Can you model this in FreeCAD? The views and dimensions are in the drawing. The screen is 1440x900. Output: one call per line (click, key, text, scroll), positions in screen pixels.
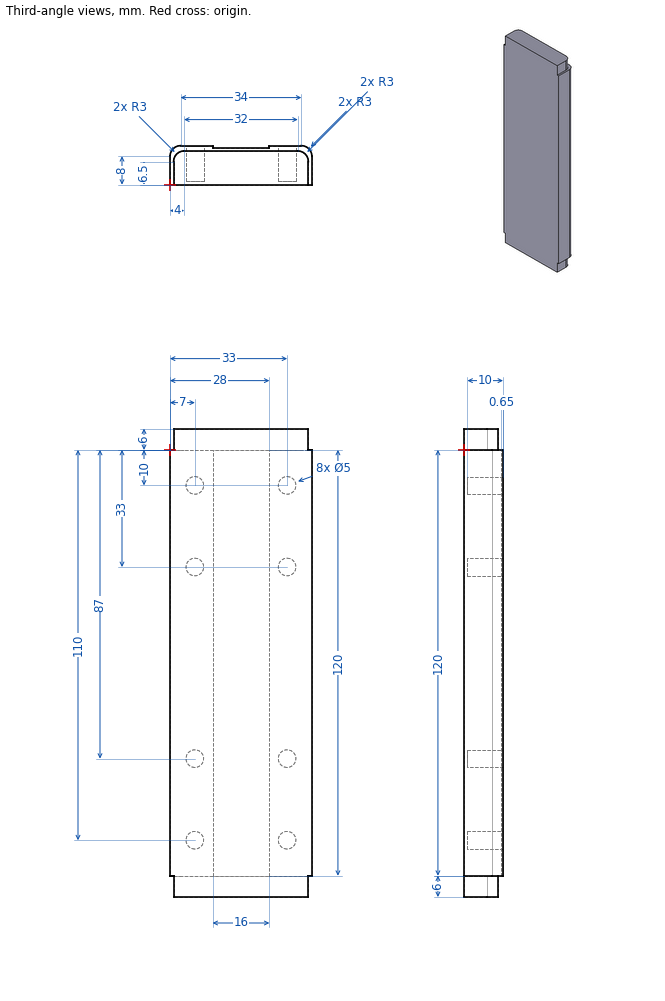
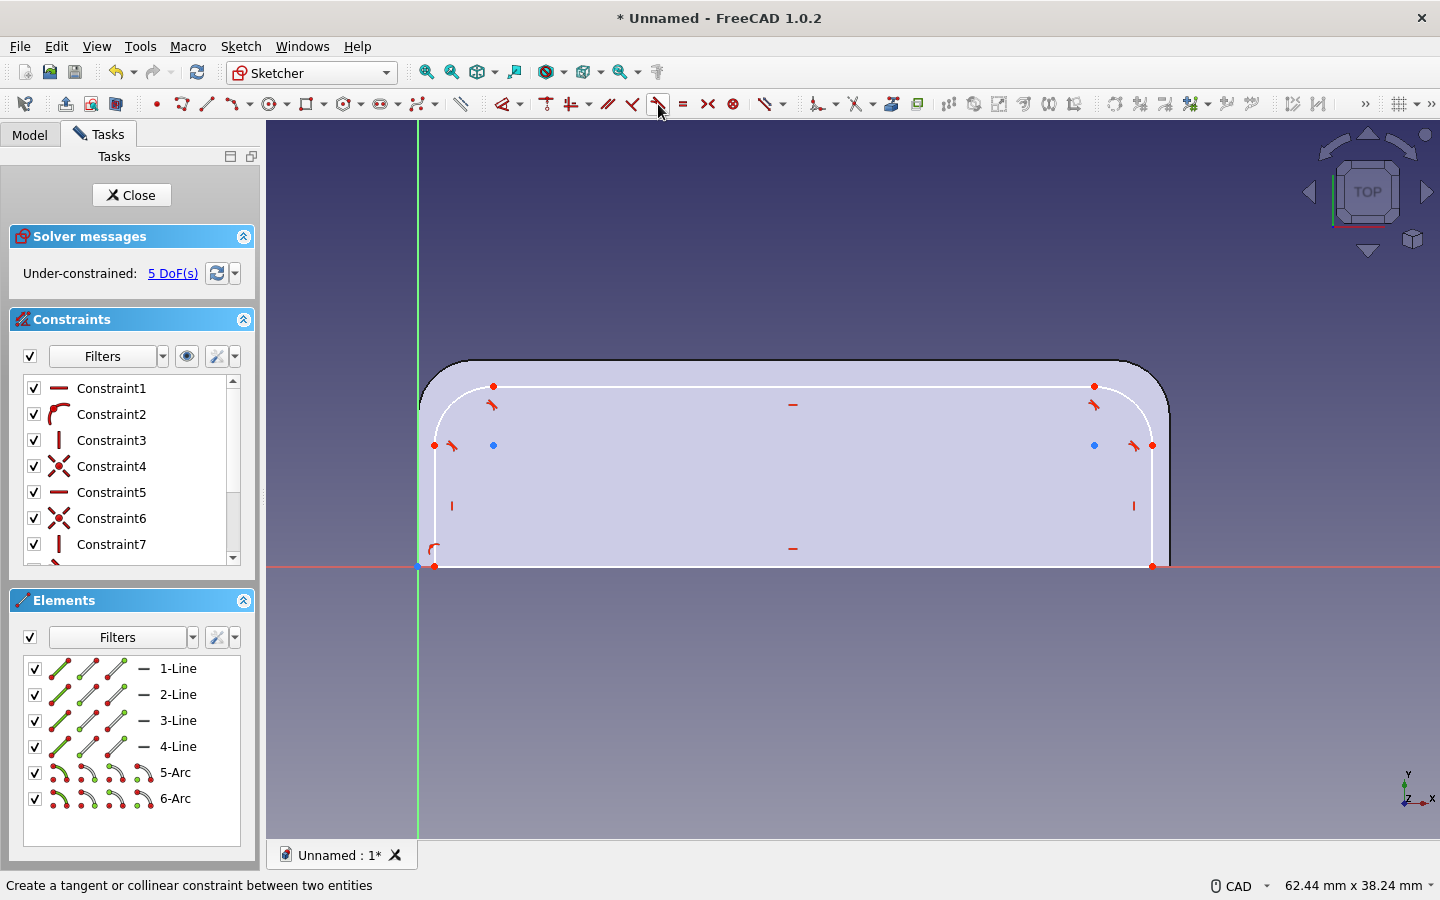
click(467, 393)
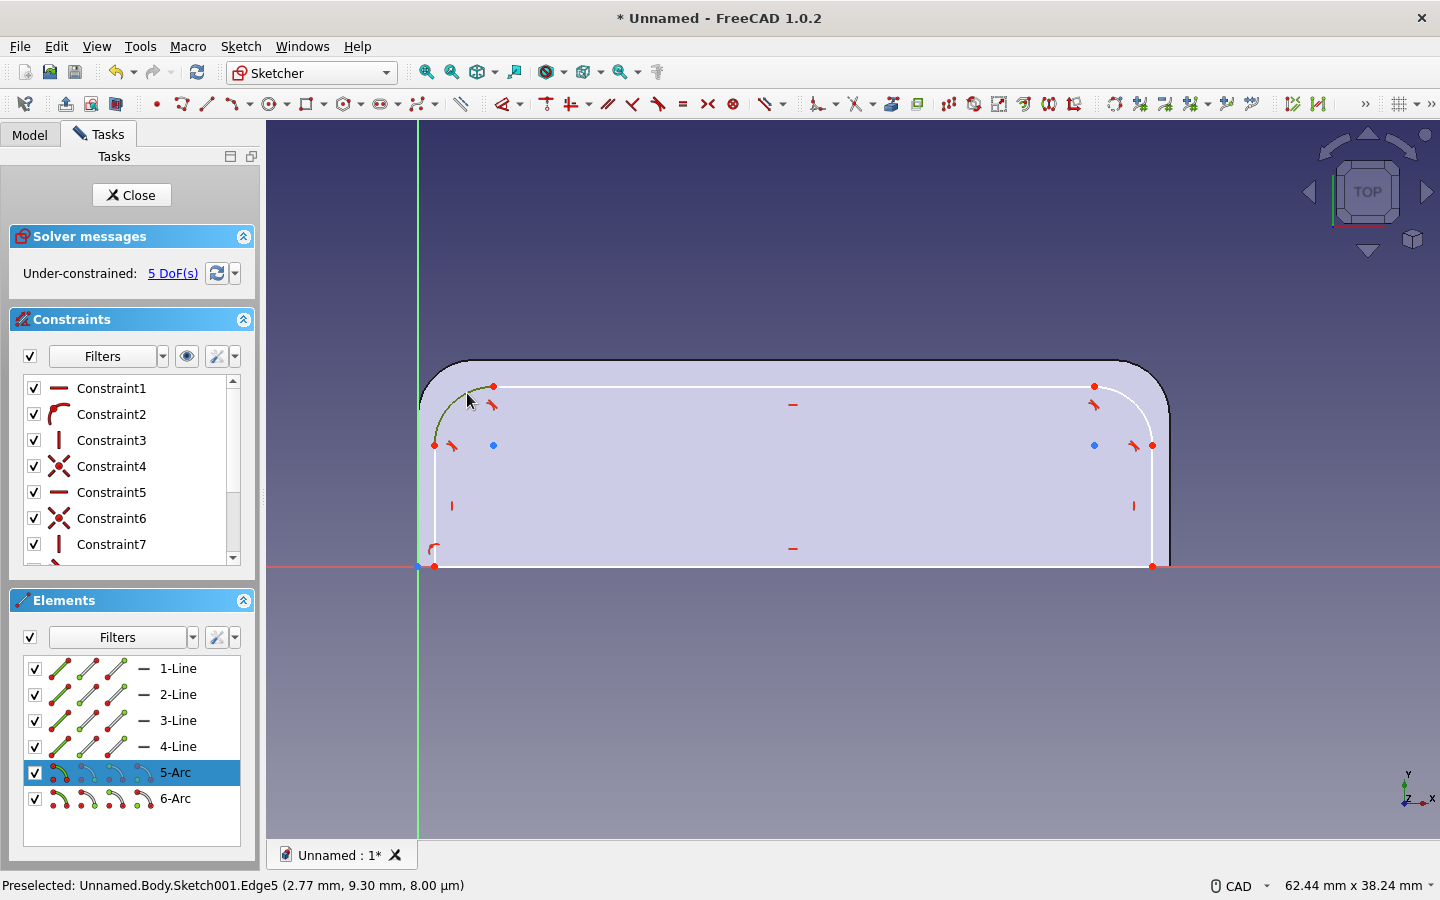
click(1146, 419)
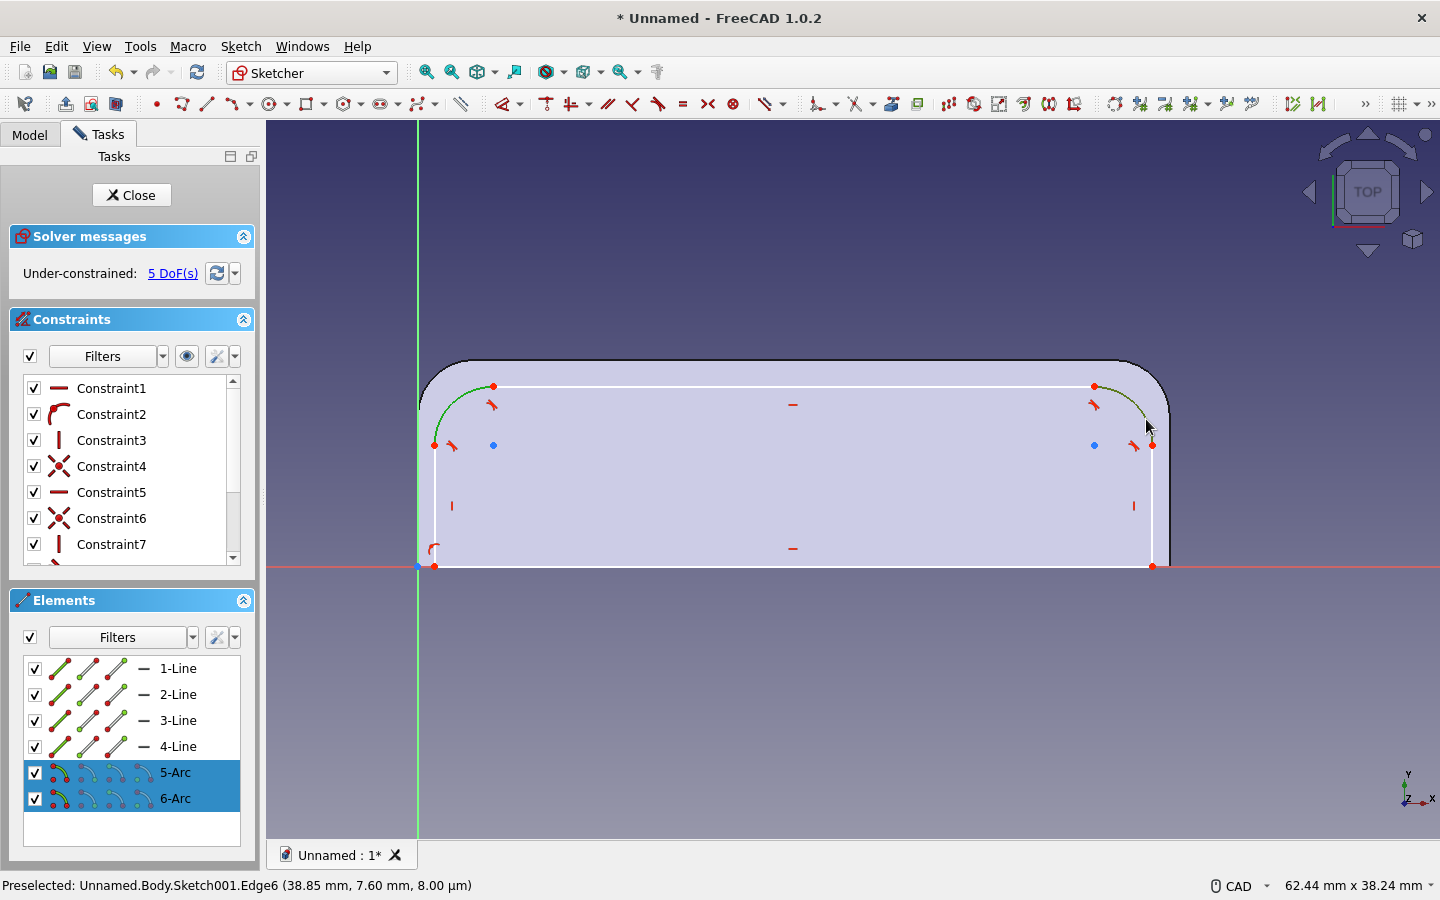
click(683, 104)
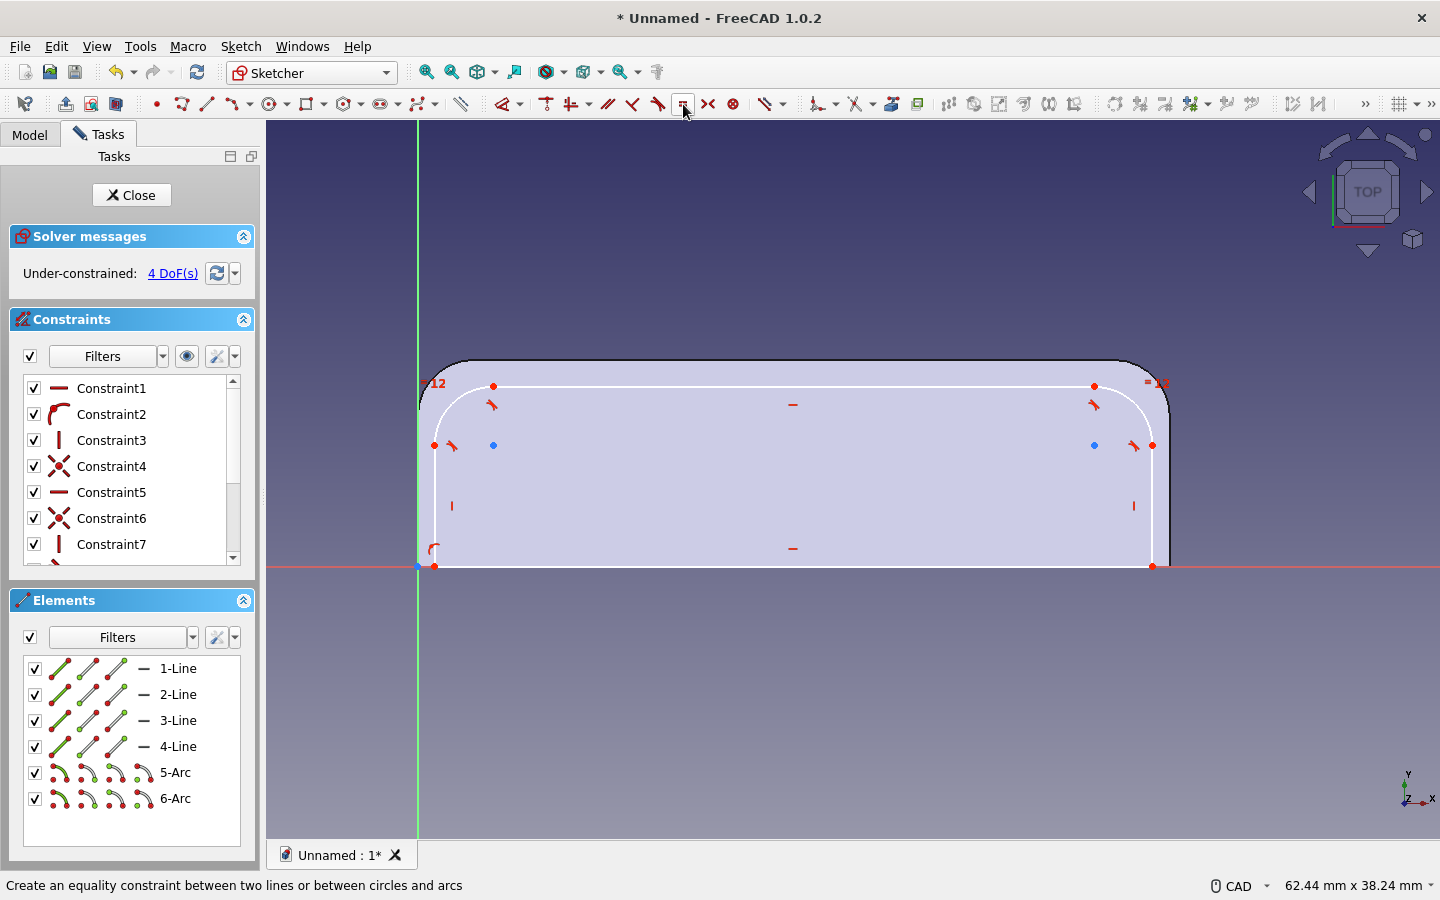
key(d)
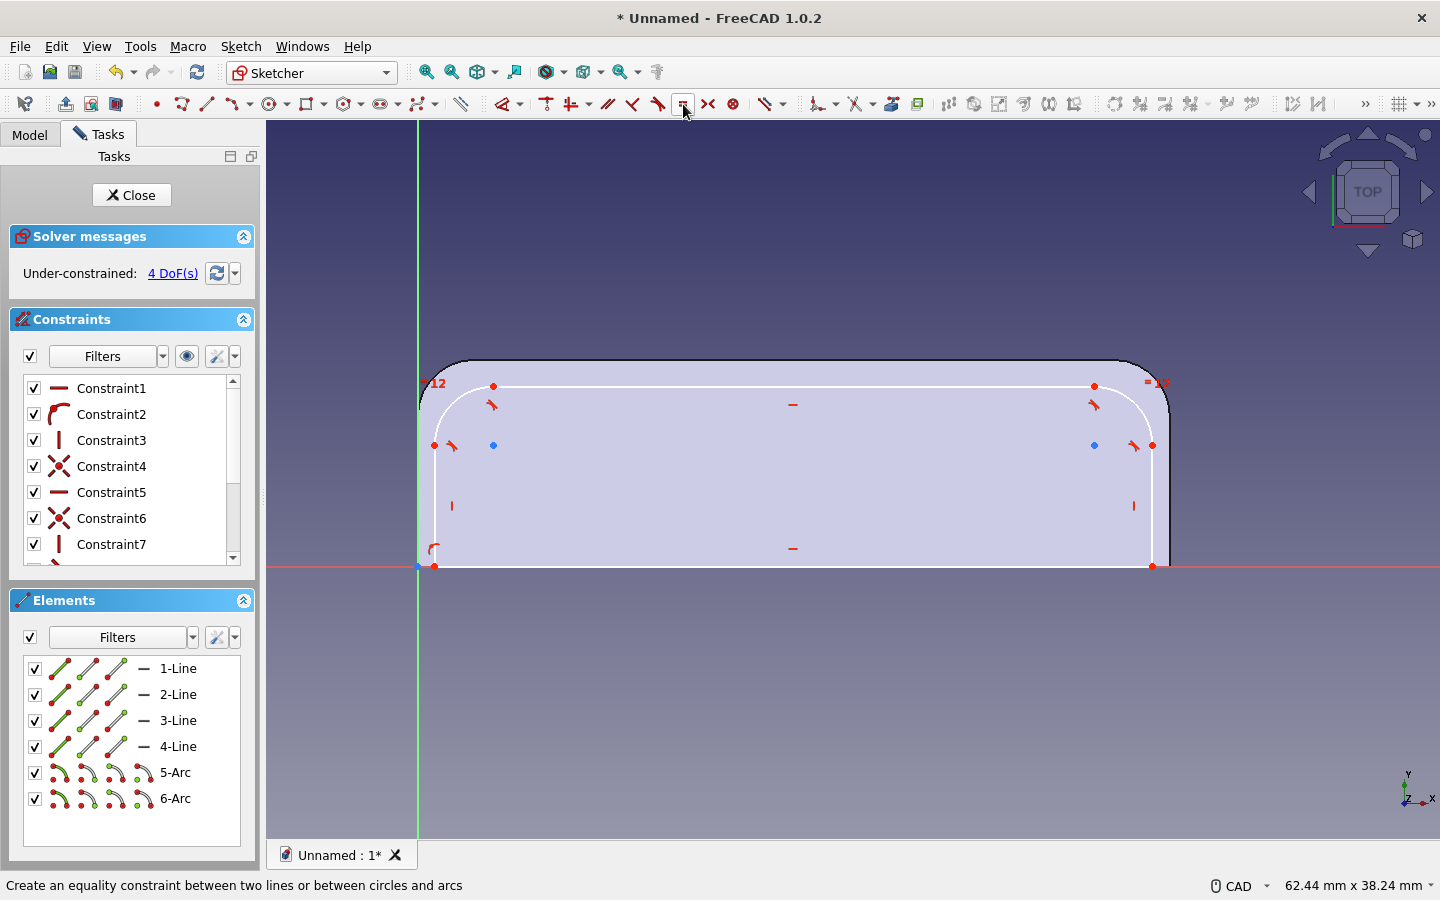
click(467, 393)
click(453, 364)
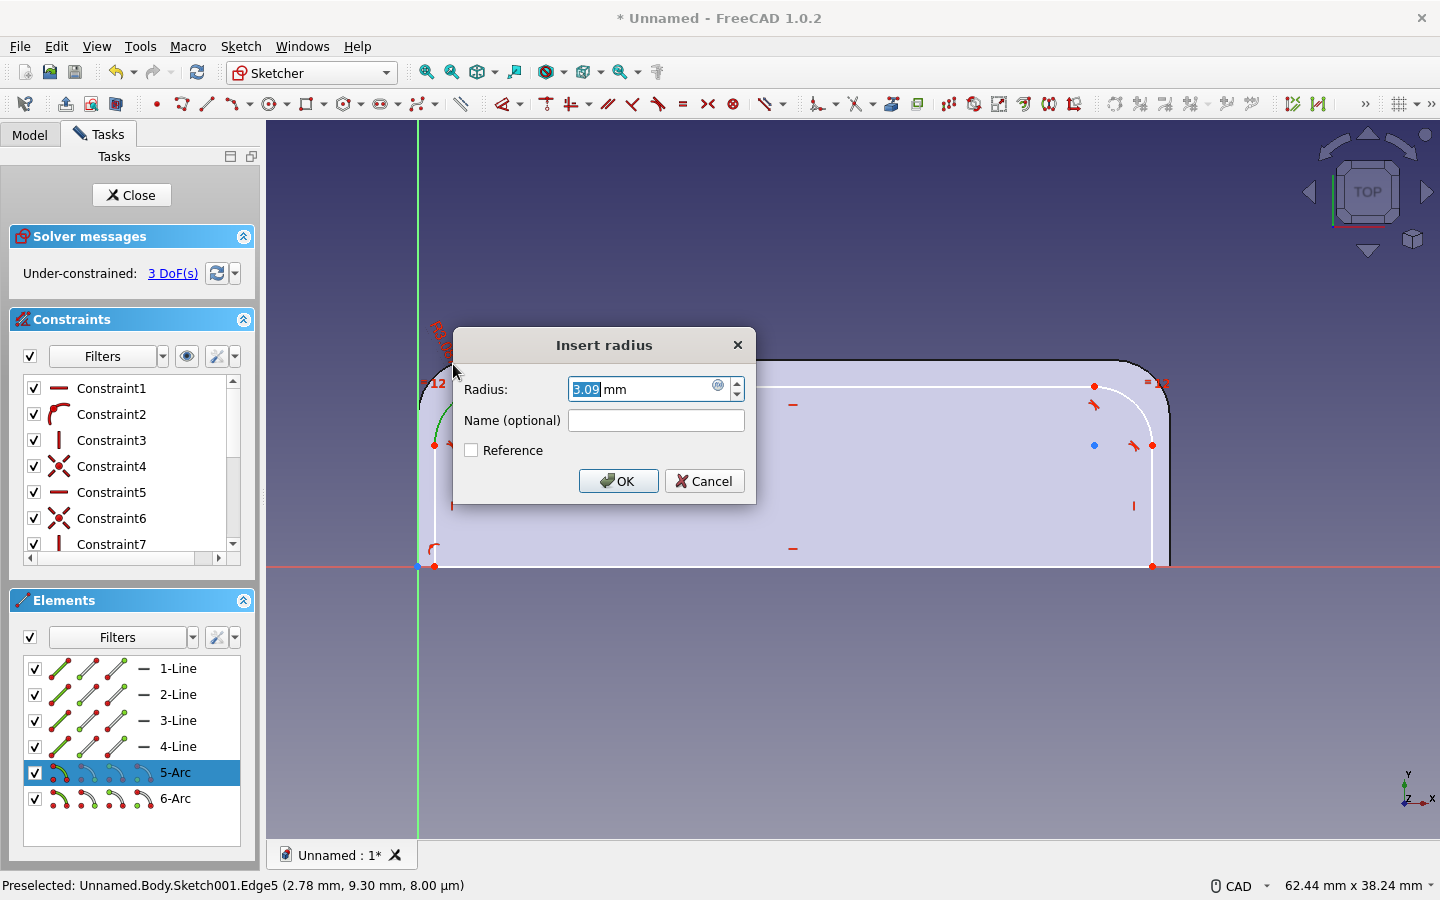
text(3)
key(Return)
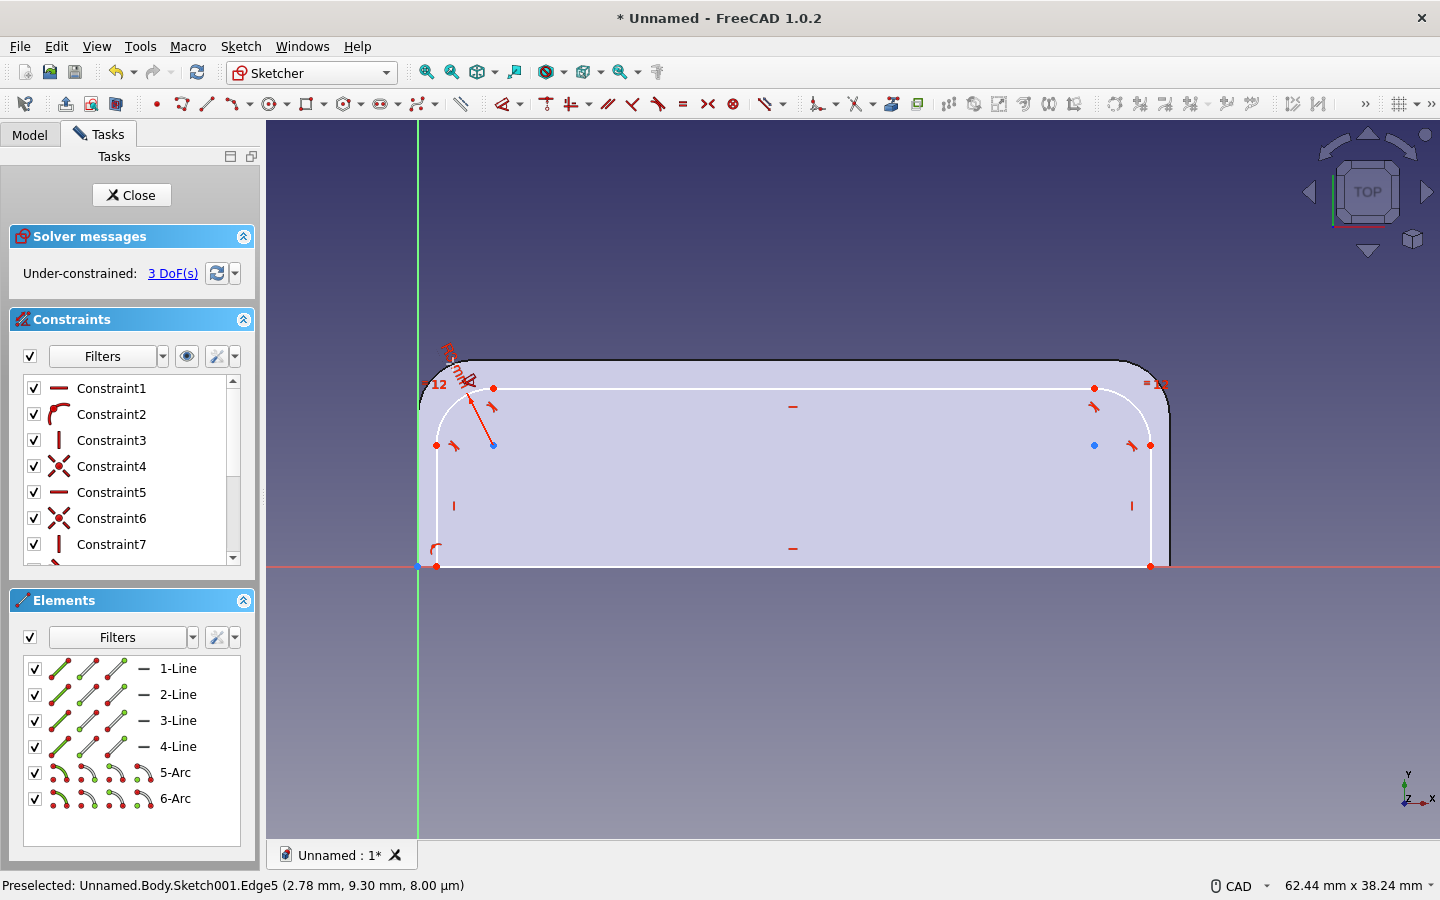
click(914, 389)
click(794, 355)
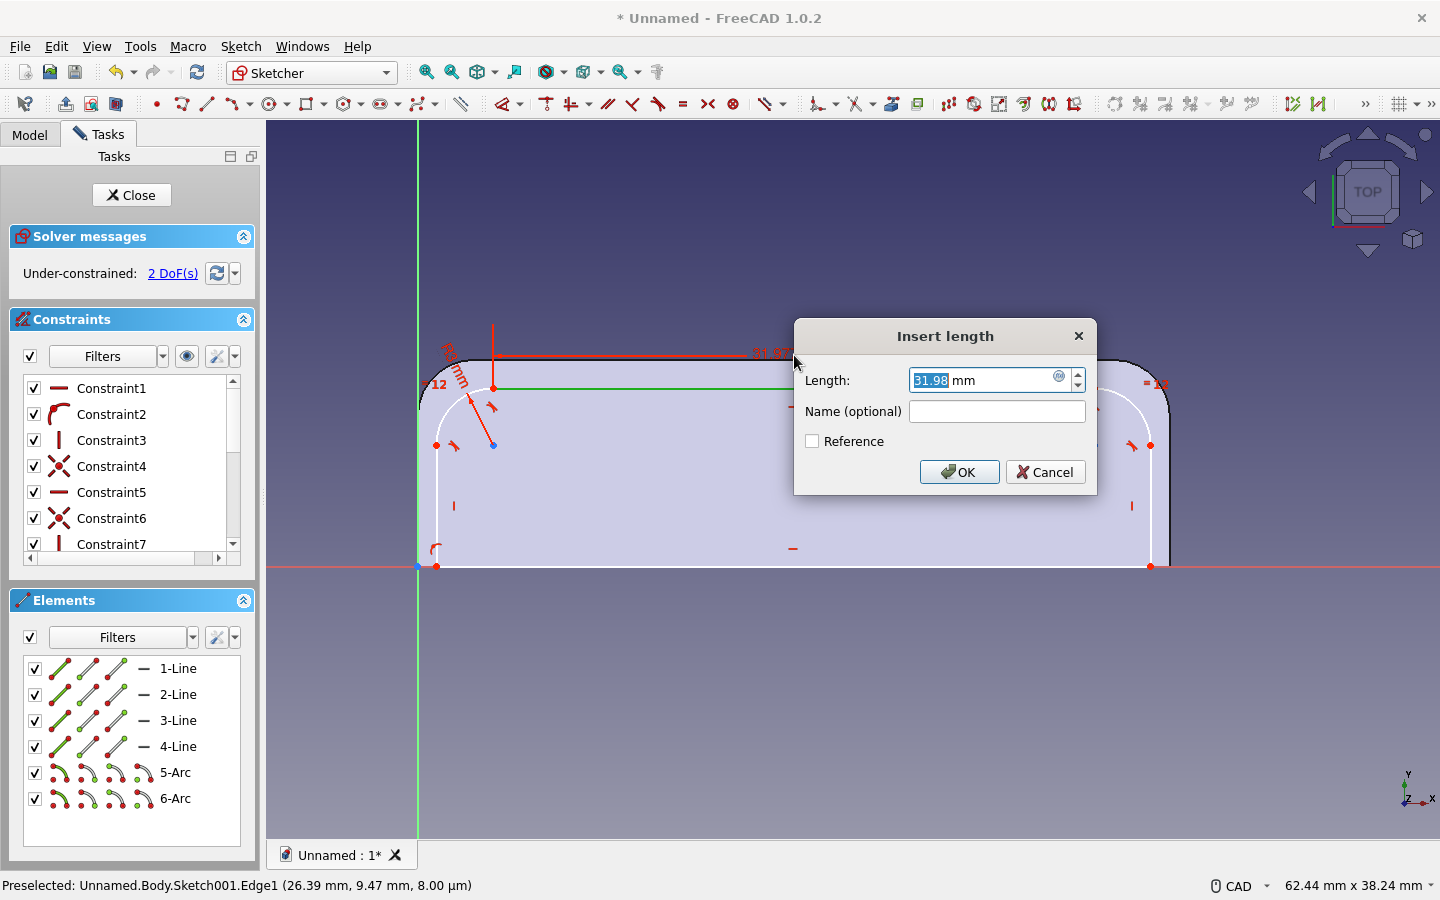
text(32)
key(Return)